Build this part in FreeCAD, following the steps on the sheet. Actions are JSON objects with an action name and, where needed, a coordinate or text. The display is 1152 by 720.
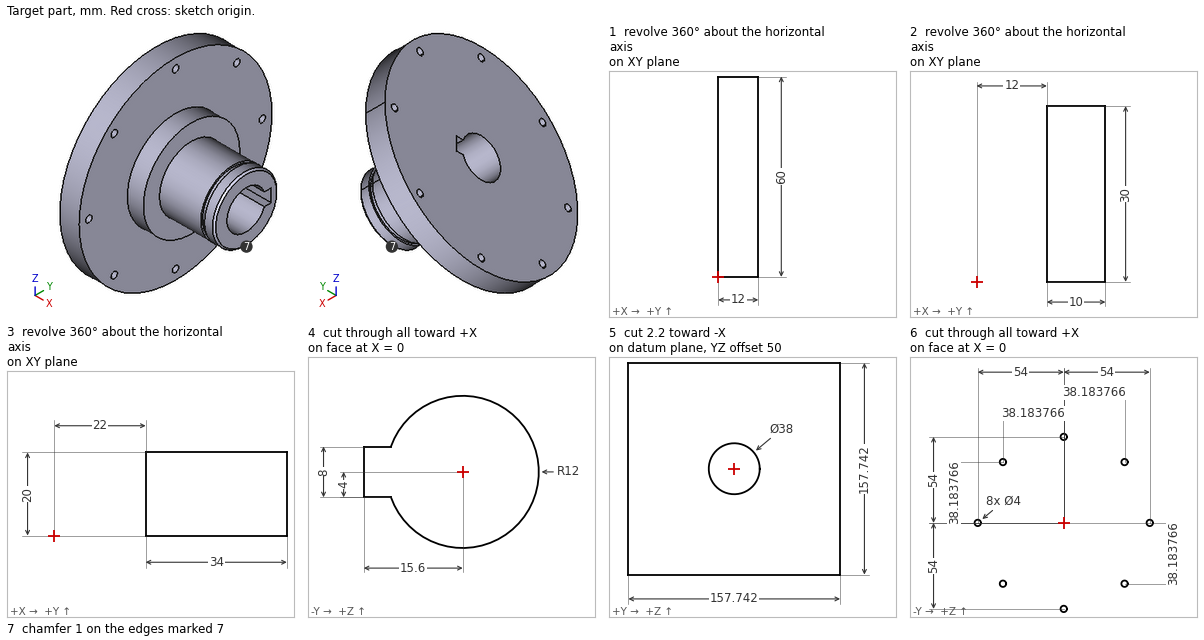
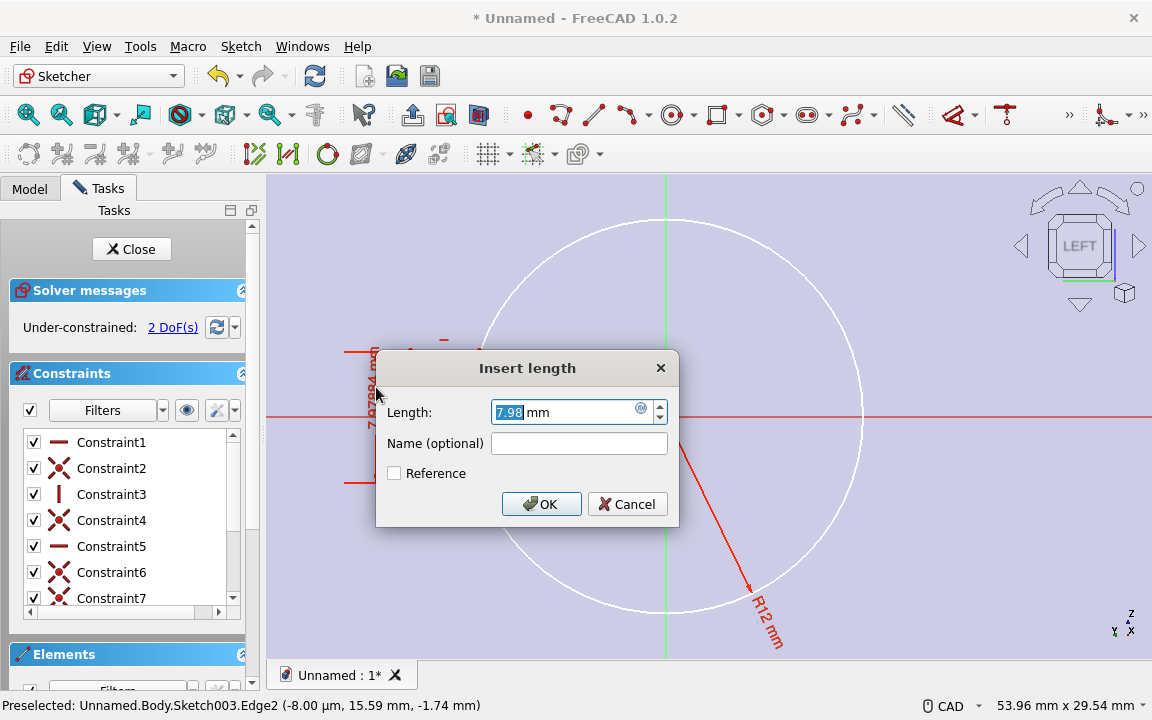
{"action": "type", "text": "8"}
{"action": "key", "text": "Return"}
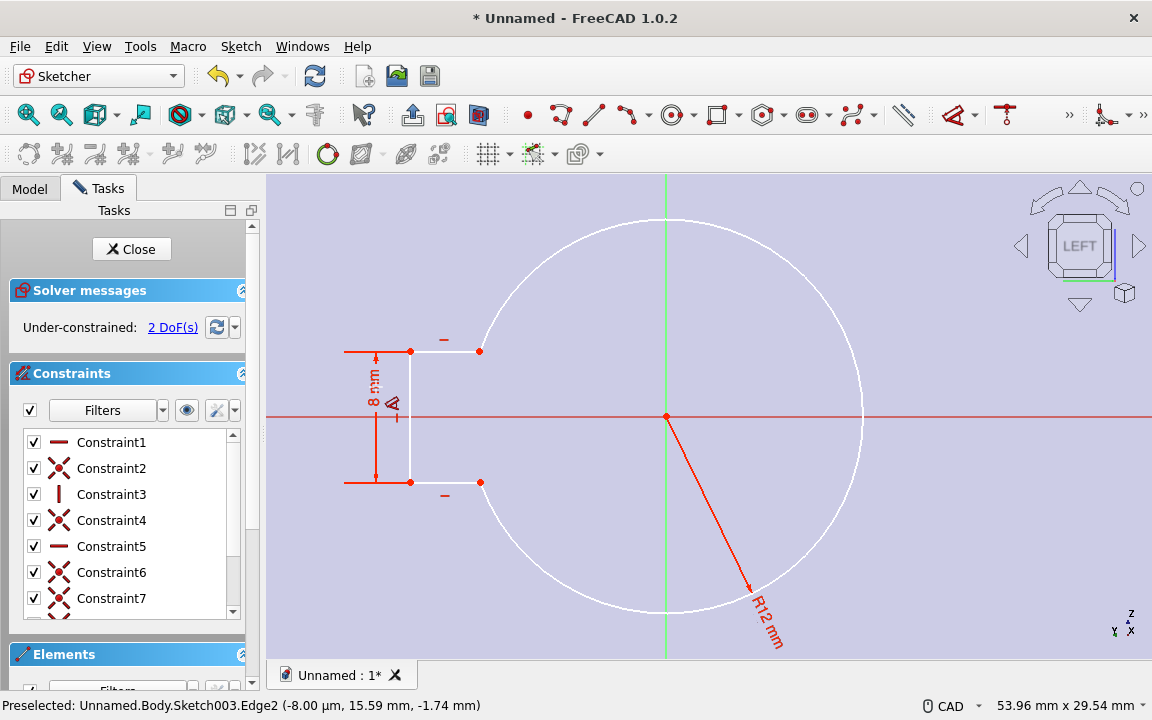
{"action": "left_click", "coordinate": [481, 483]}
{"action": "left_click", "coordinate": [447, 450]}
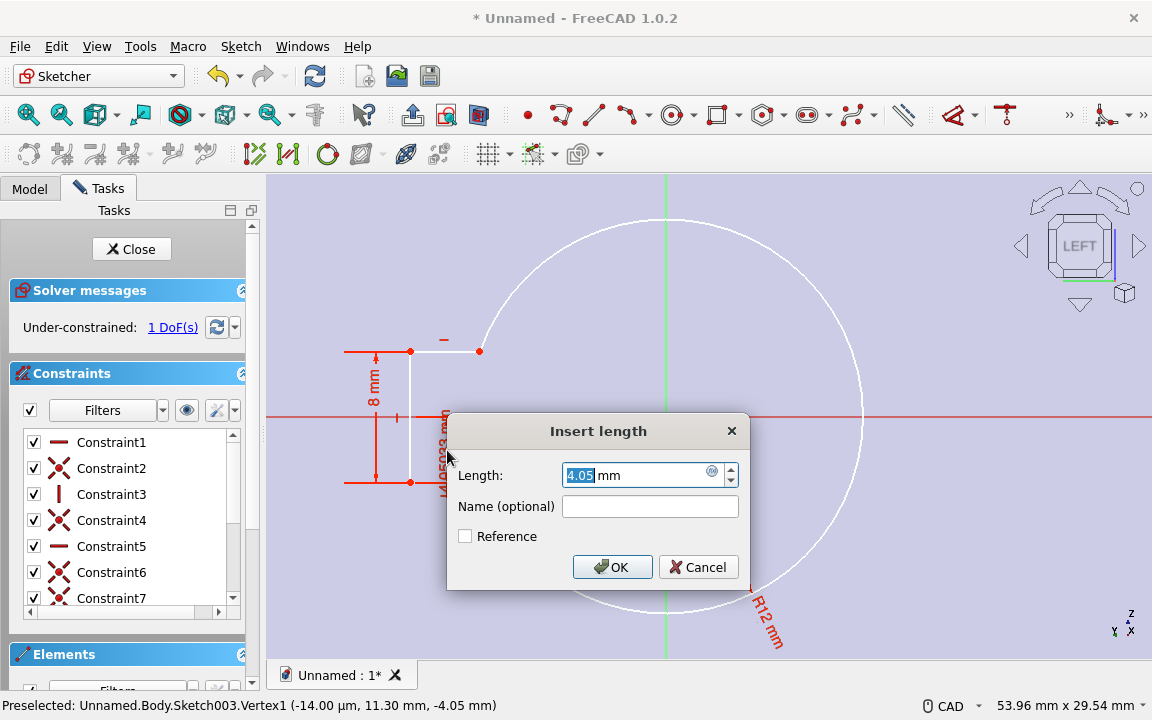
{"action": "type", "text": "4"}
{"action": "key", "text": "Return"}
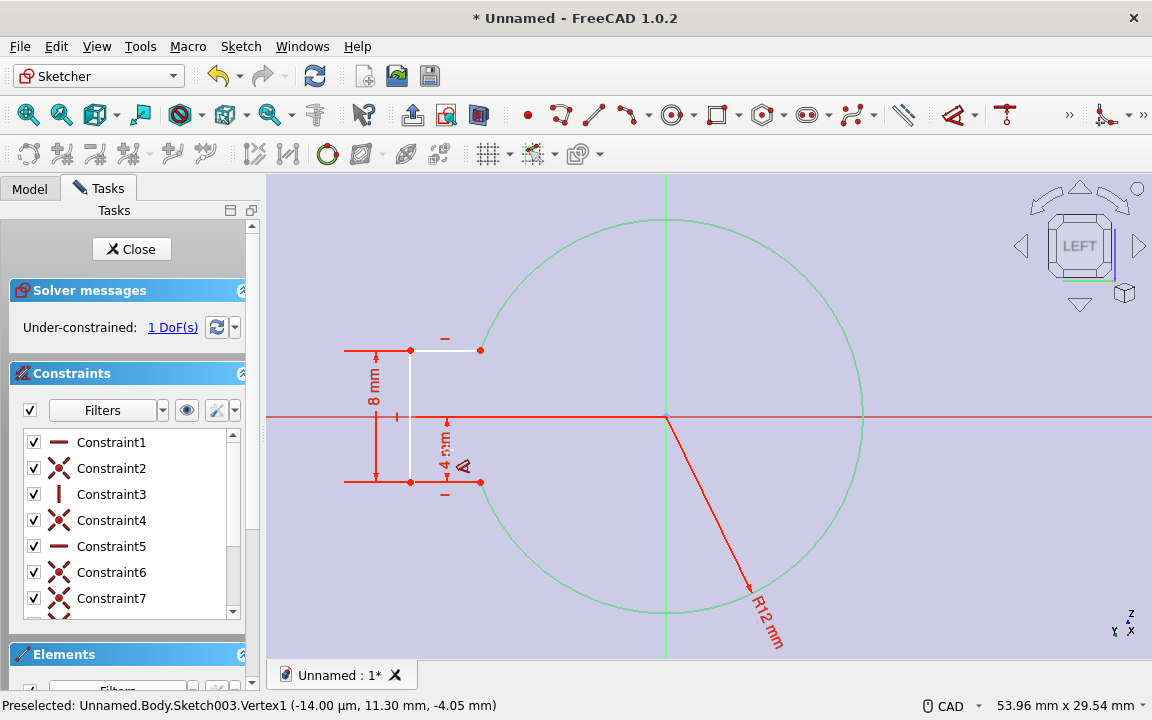
{"action": "left_click", "coordinate": [410, 482]}
{"action": "left_click", "coordinate": [538, 516]}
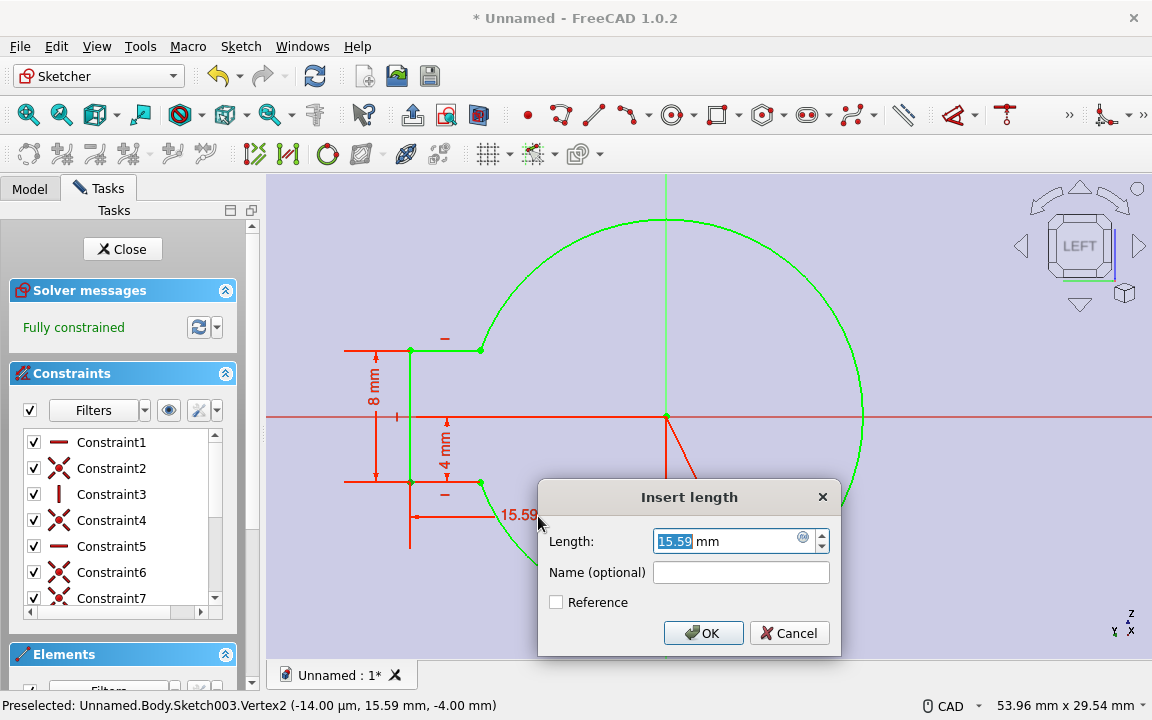
{"action": "type", "text": "15.6"}
{"action": "key", "text": "Return"}
{"action": "key", "text": "Escape"}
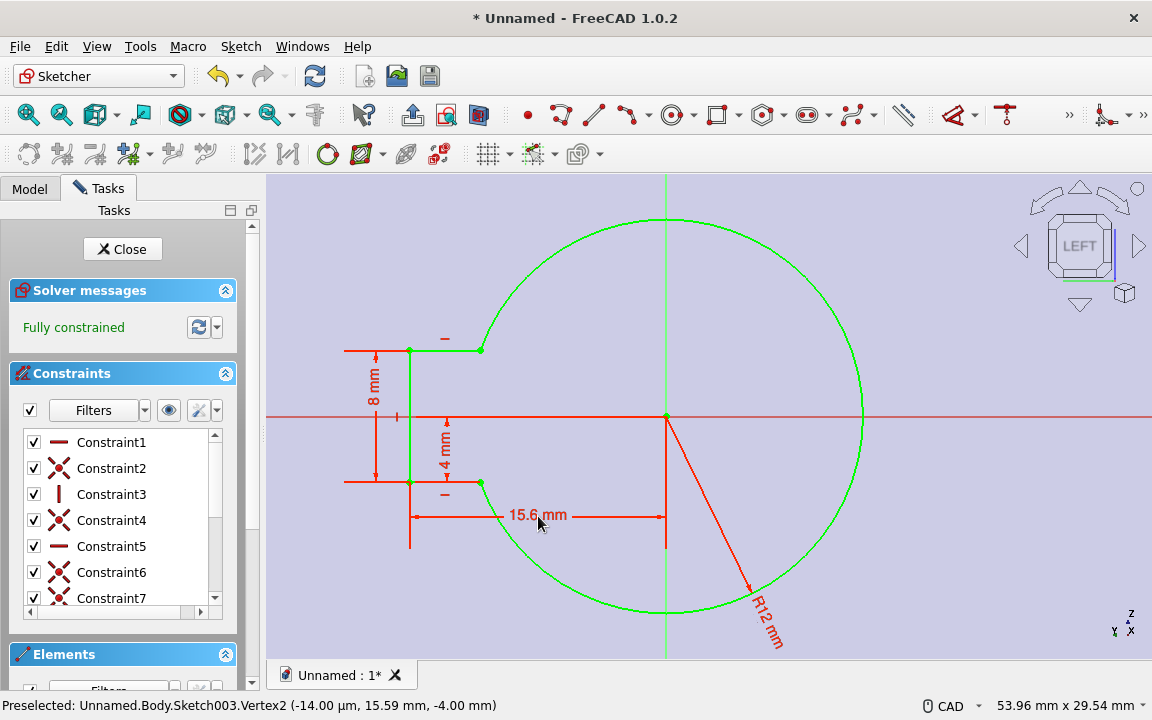
{"action": "left_click", "coordinate": [123, 249]}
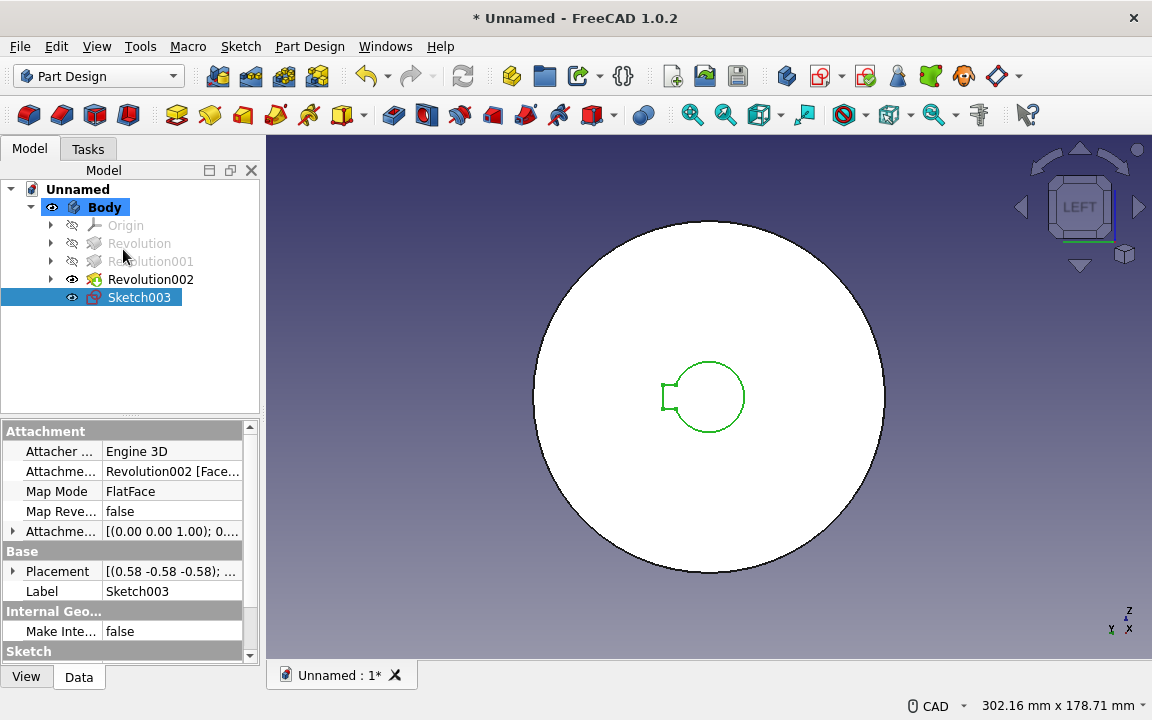
{"action": "left_click", "coordinate": [394, 116]}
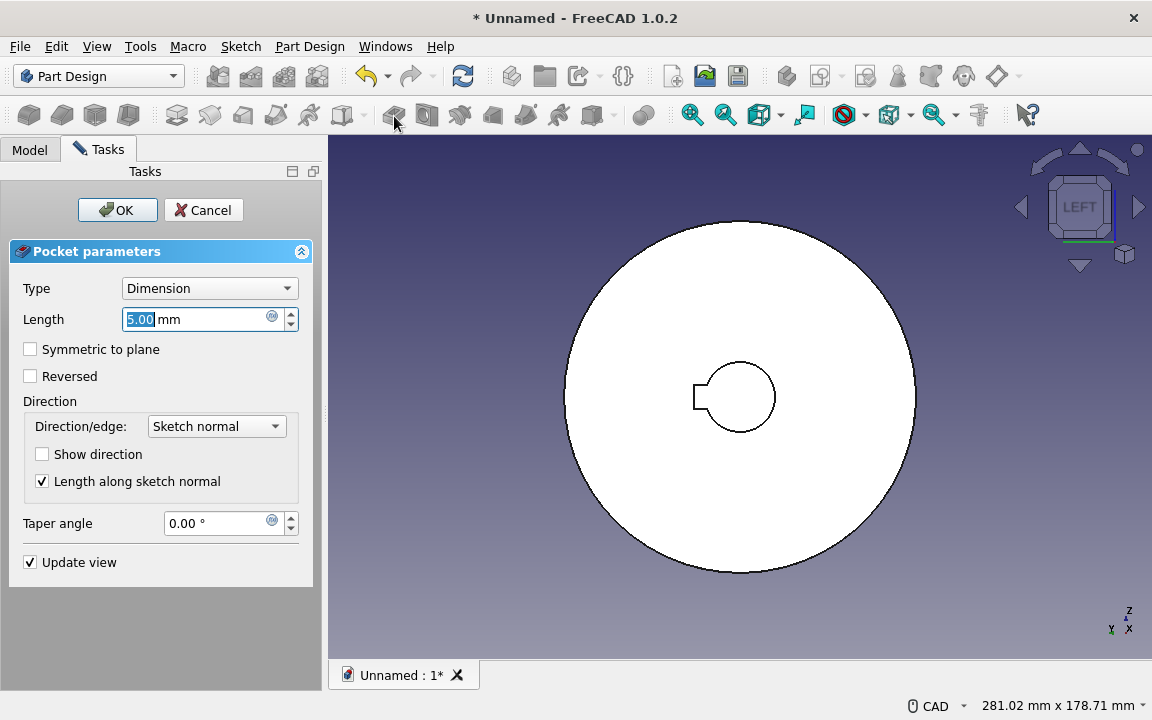
{"action": "left_click", "coordinate": [210, 288]}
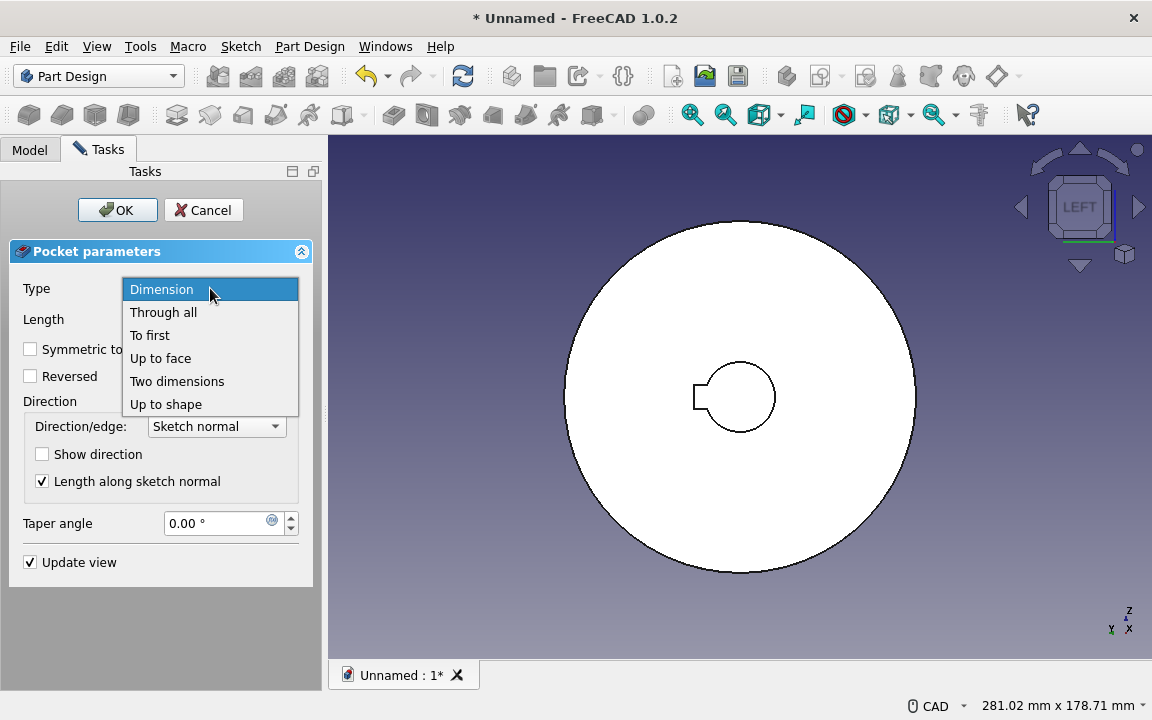
{"action": "left_click", "coordinate": [208, 312]}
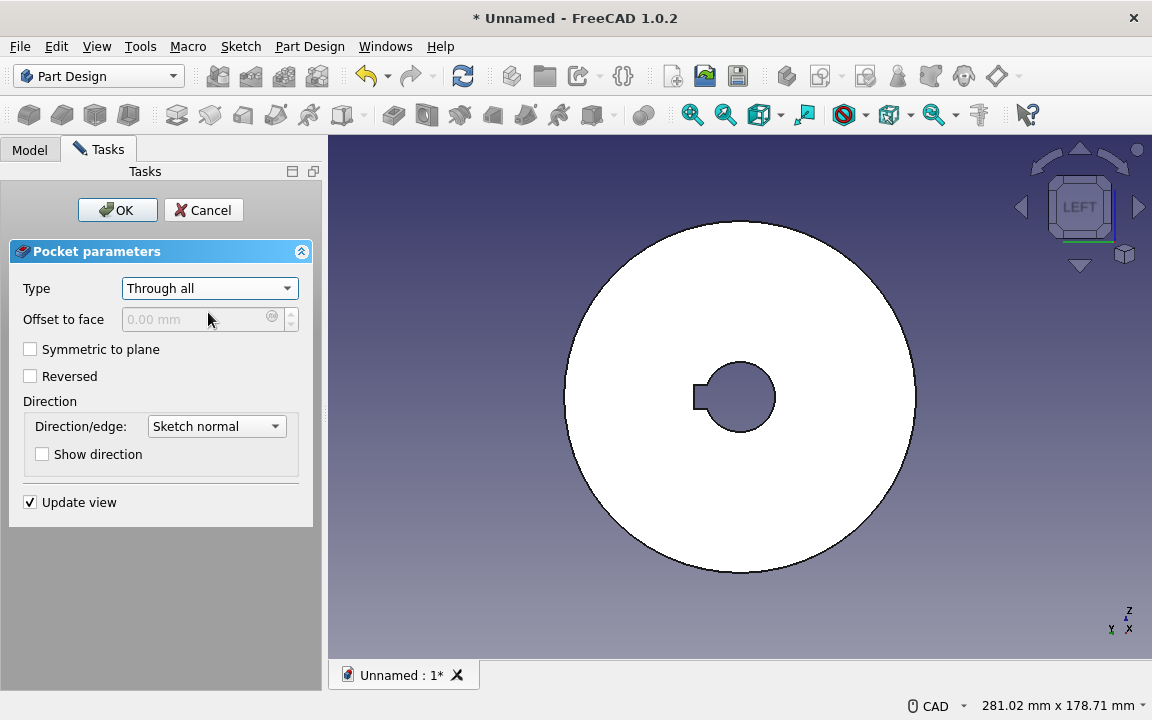
{"action": "left_click", "coordinate": [118, 210]}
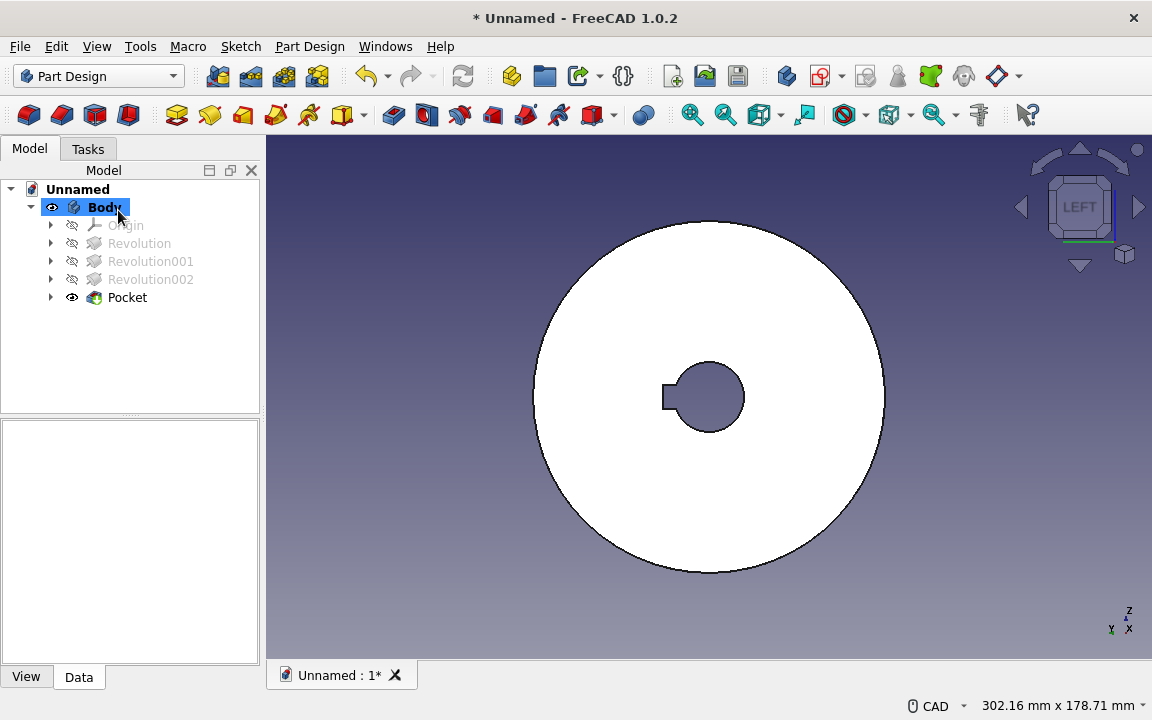
{"action": "left_click", "coordinate": [51, 225]}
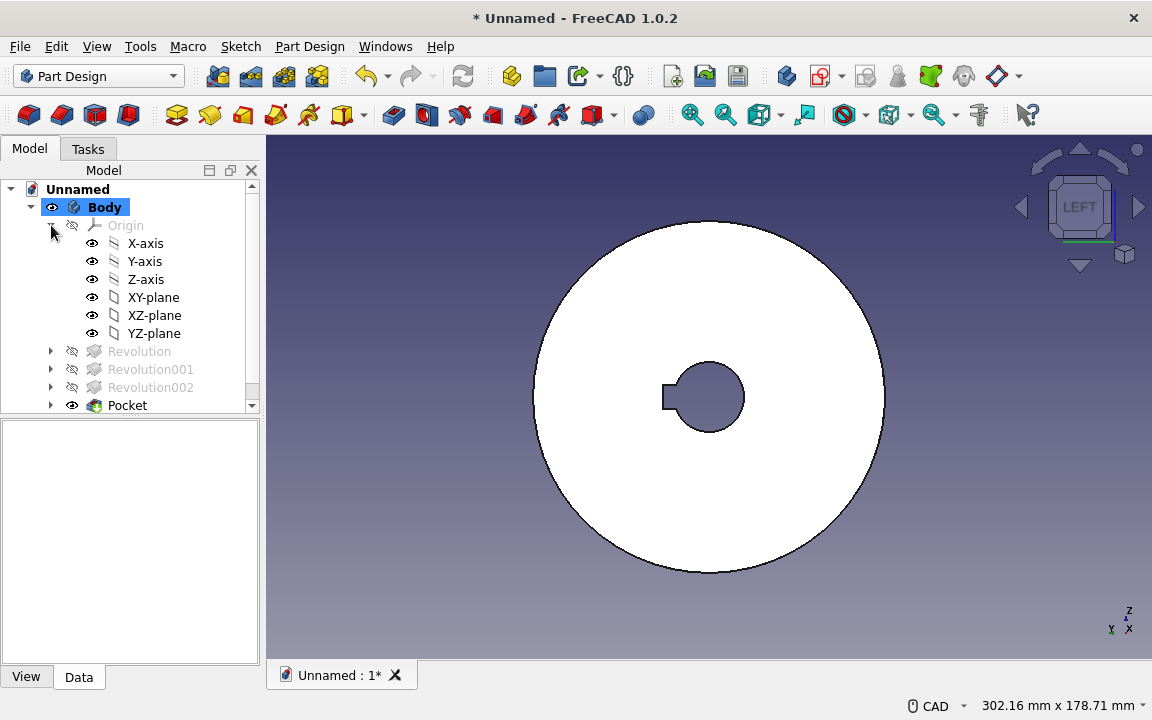
{"action": "left_click", "coordinate": [137, 333]}